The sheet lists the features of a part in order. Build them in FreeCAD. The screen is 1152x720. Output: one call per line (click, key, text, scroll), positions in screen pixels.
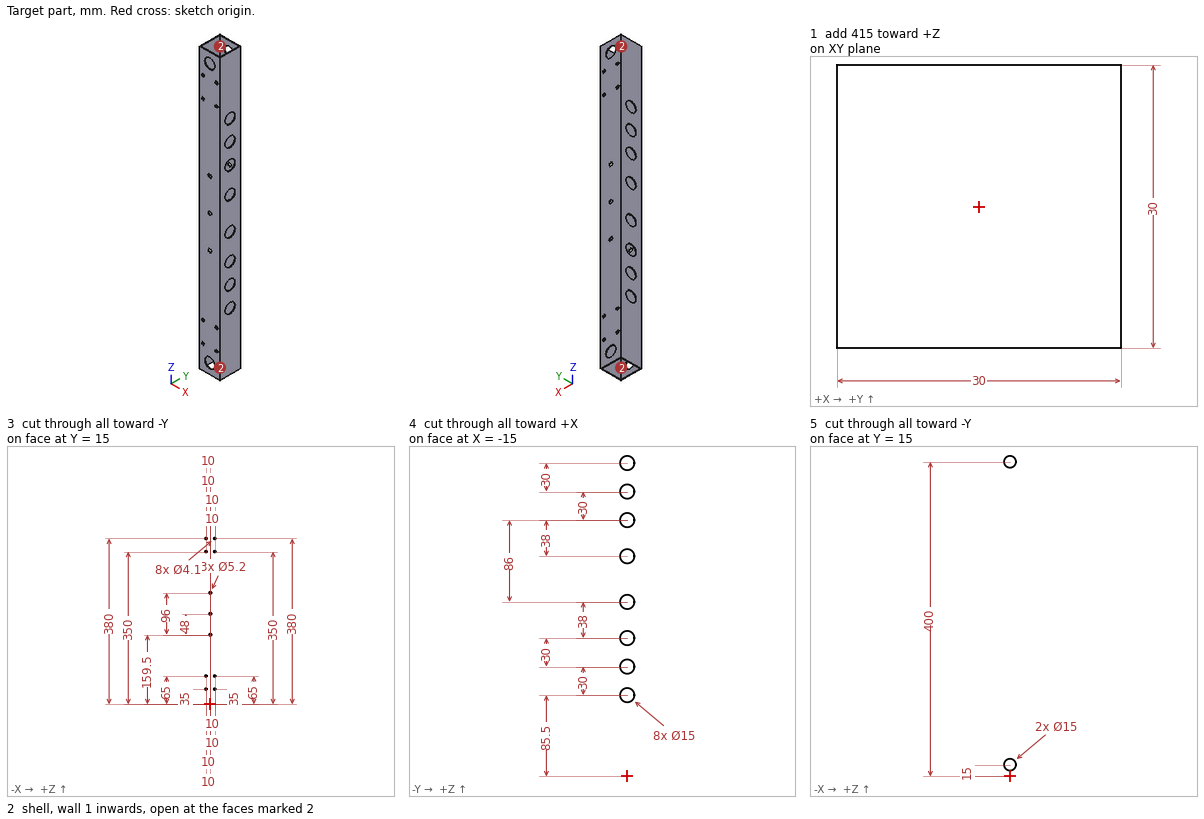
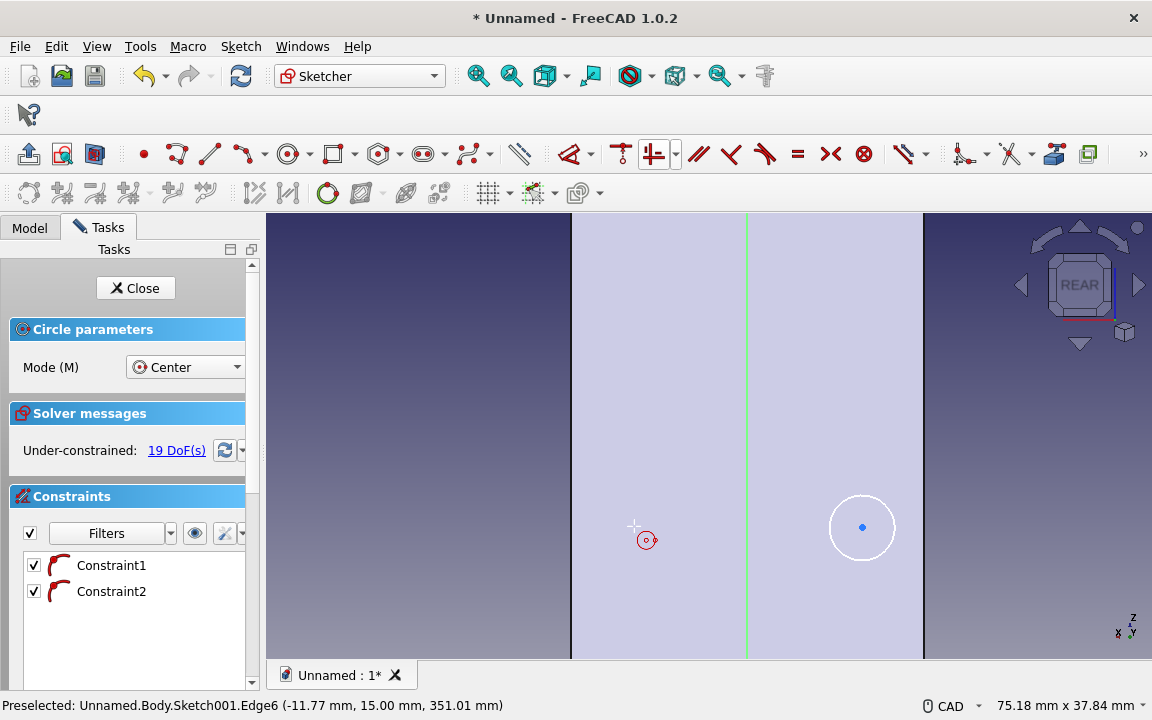
scroll(634, 527, down, 14)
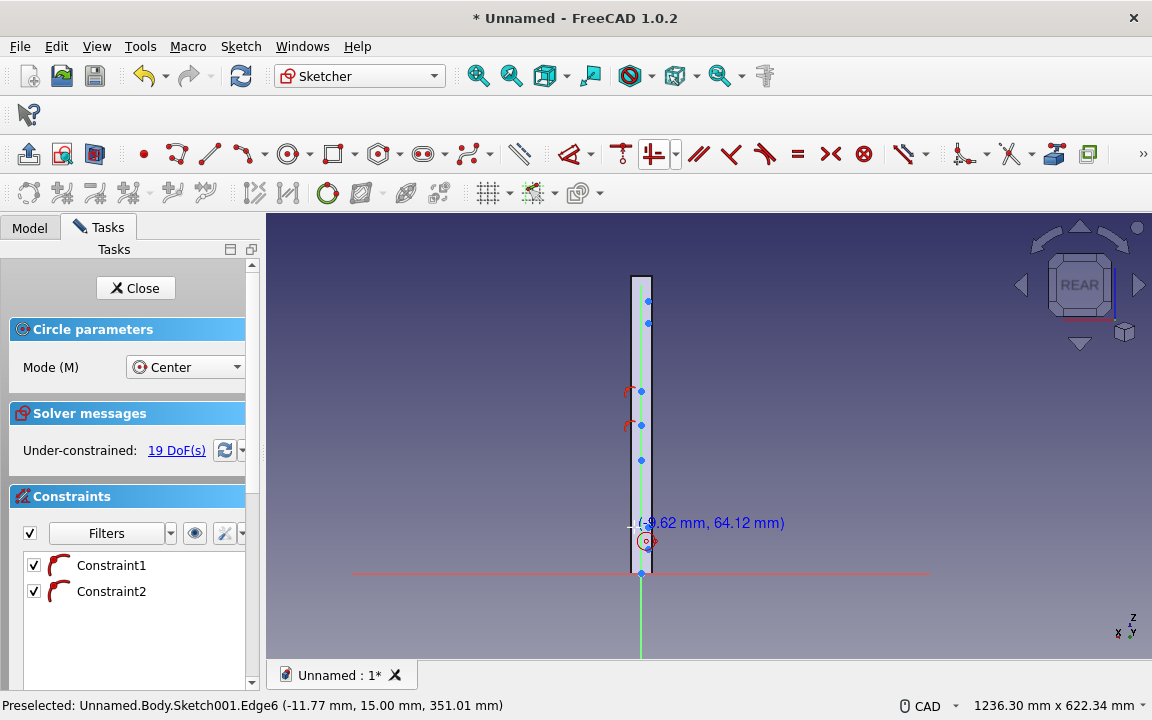
scroll(634, 527, up, 4)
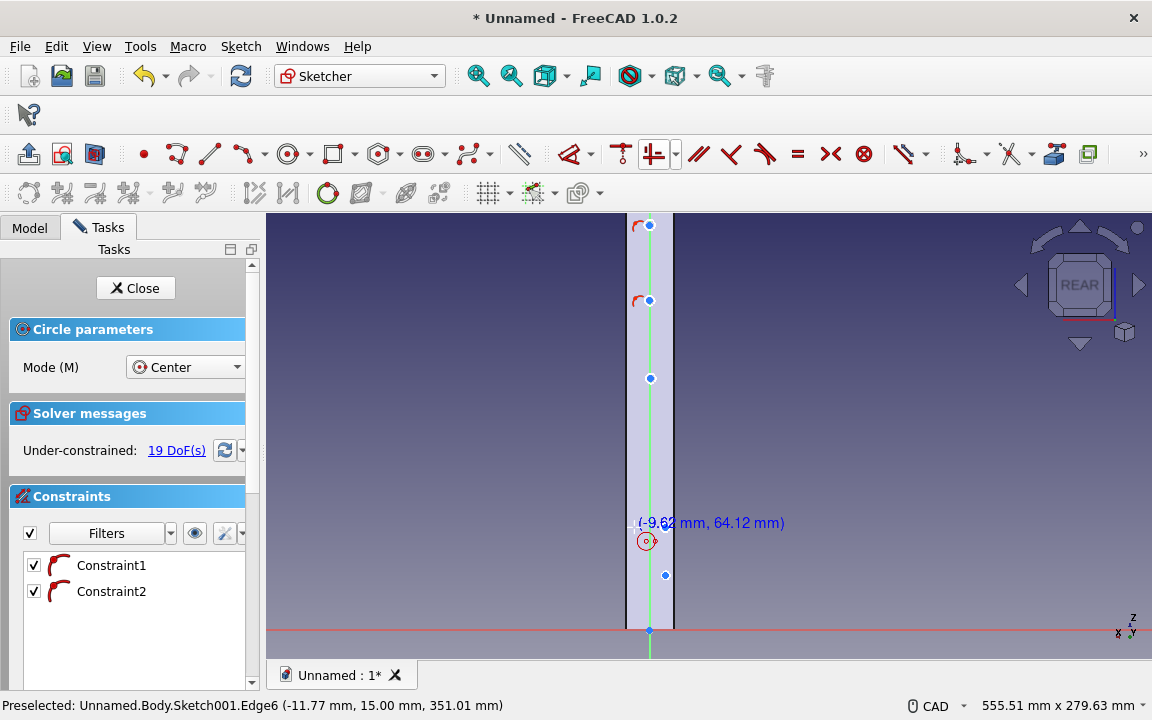
click(634, 526)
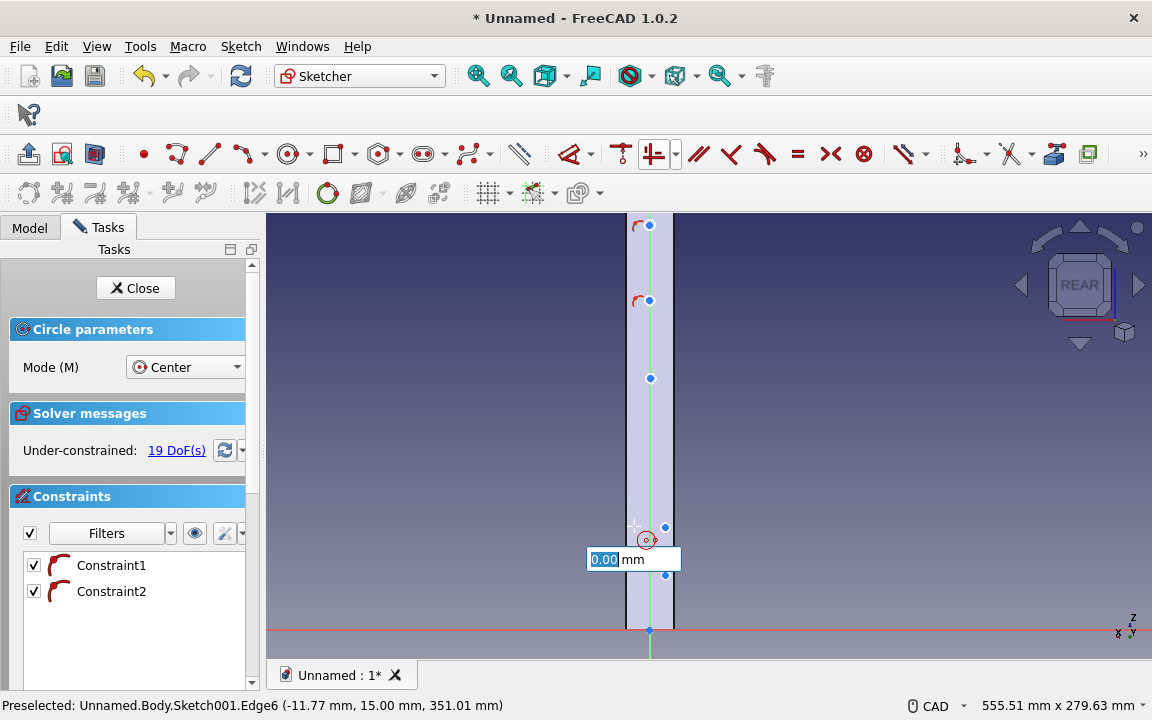
scroll(631, 524, up, 8)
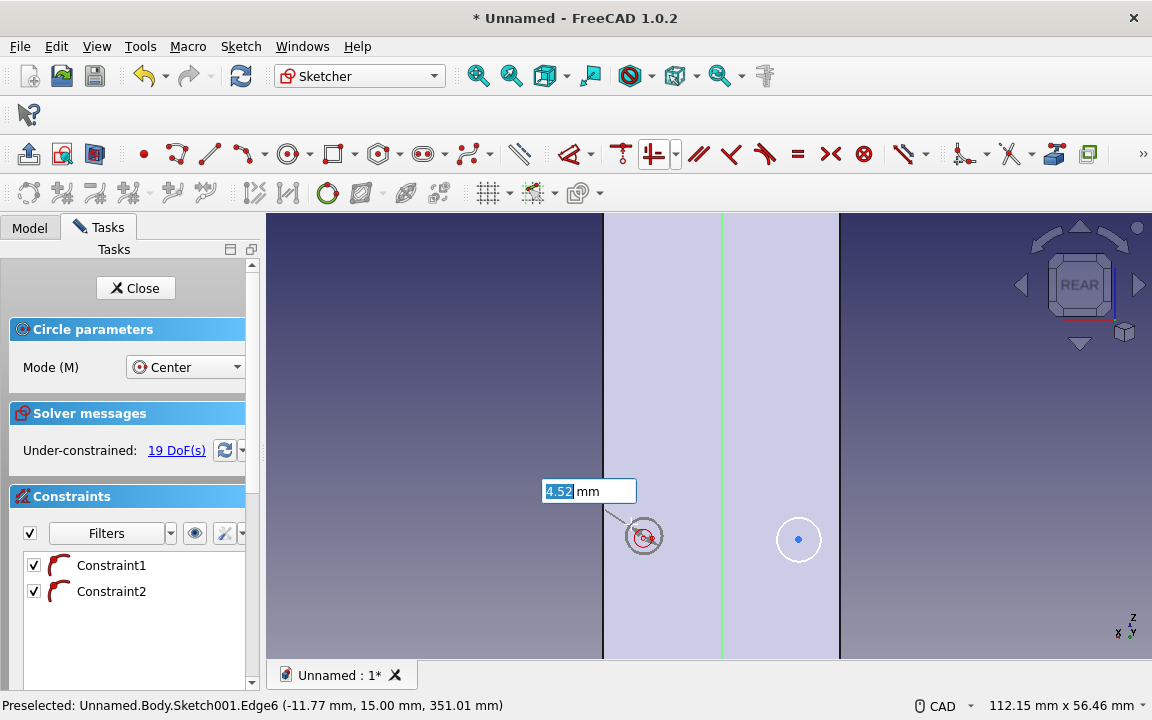
click(632, 521)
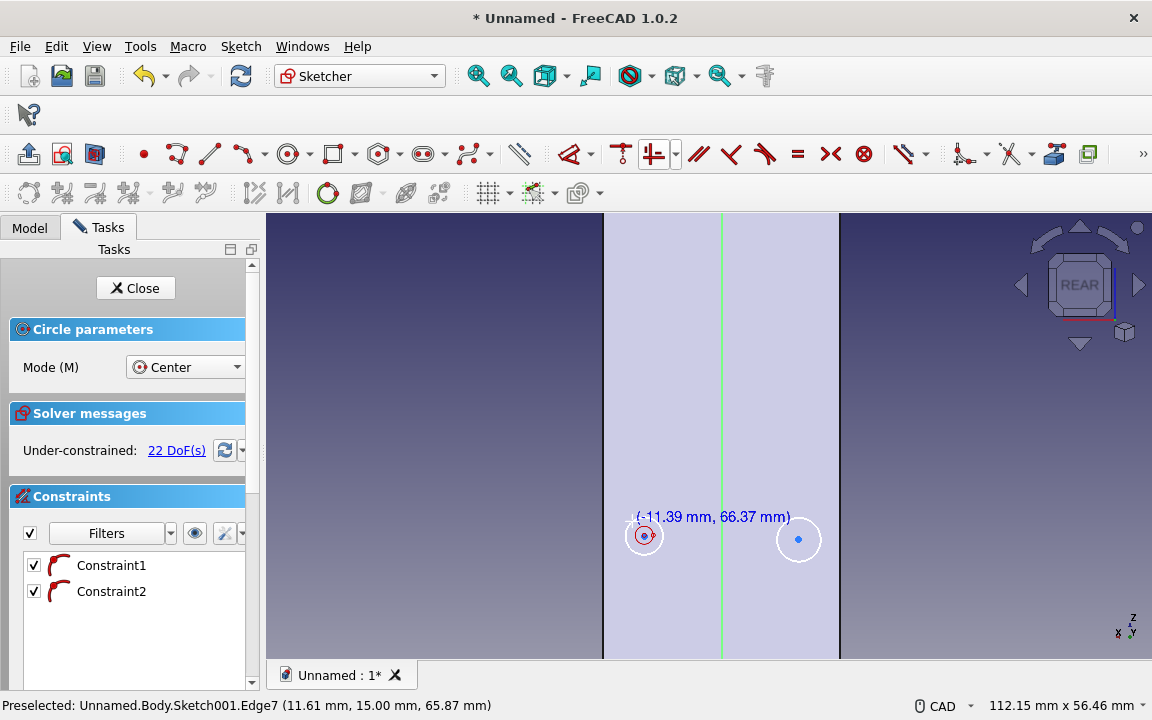
scroll(632, 526, down, 12)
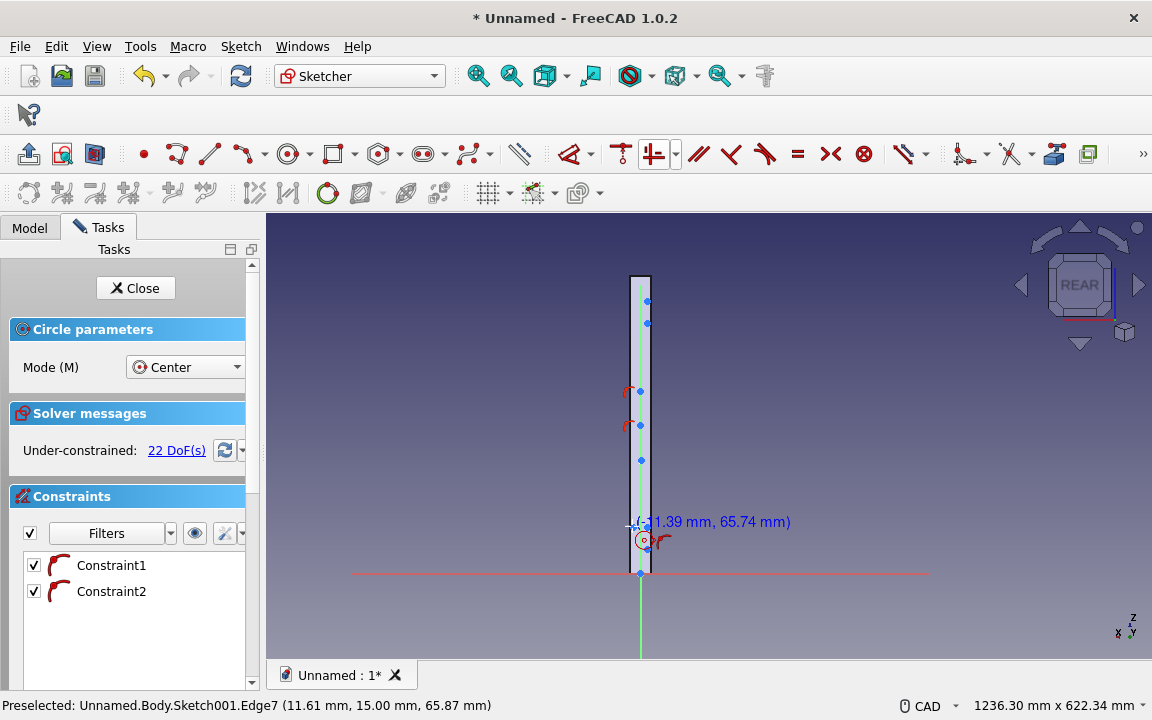
scroll(633, 323, up, 14)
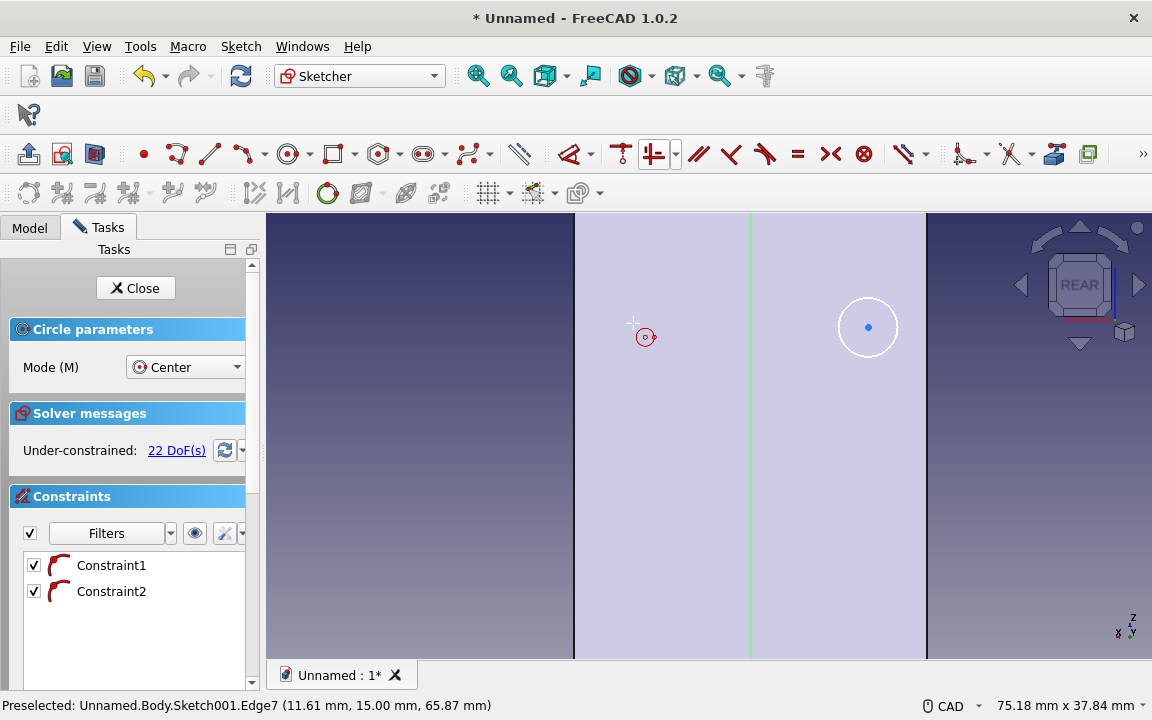
scroll(633, 322, down, 14)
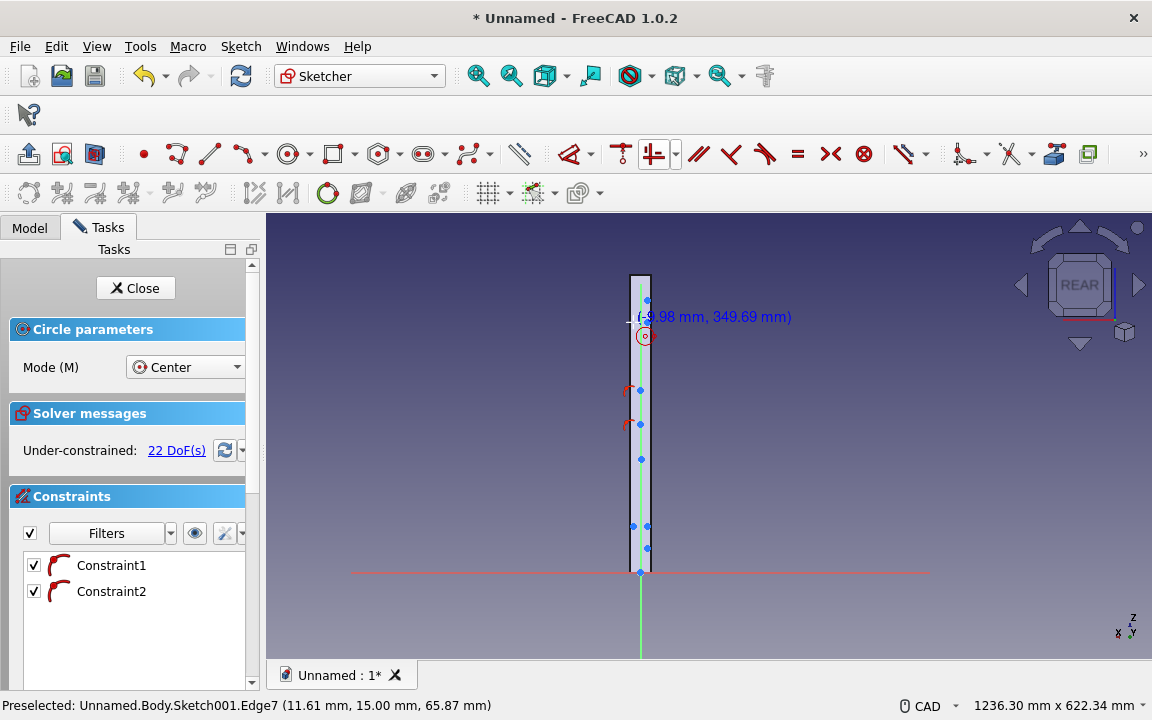
scroll(633, 322, up, 4)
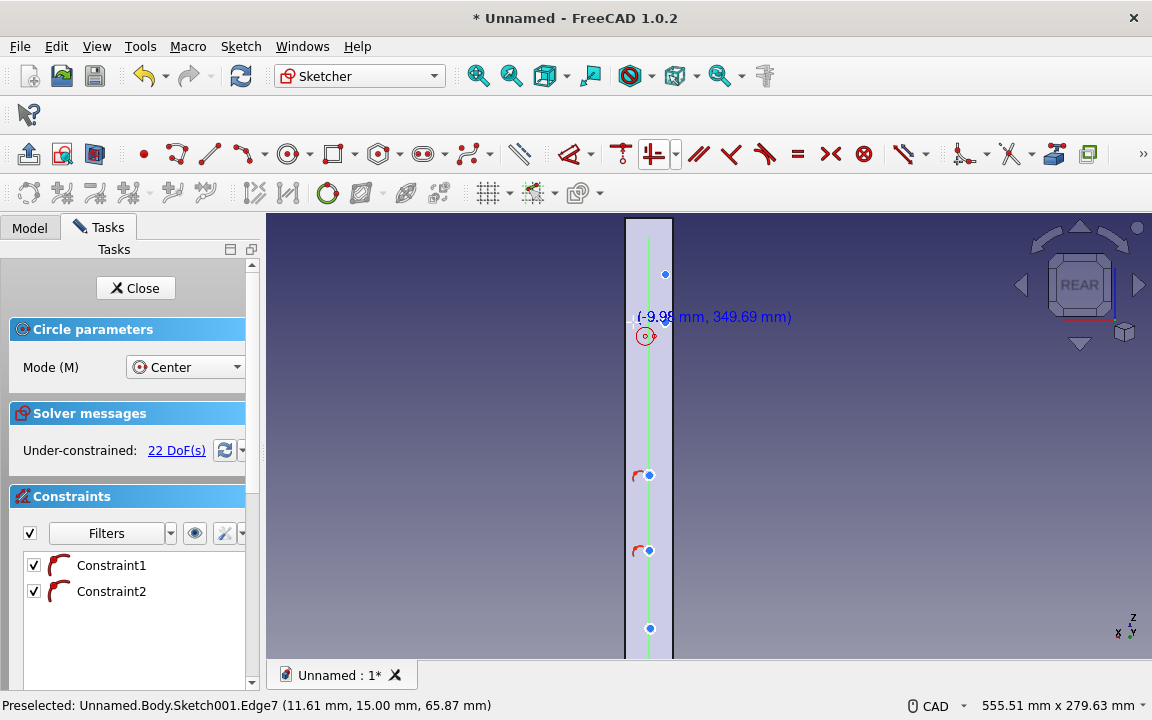
click(633, 322)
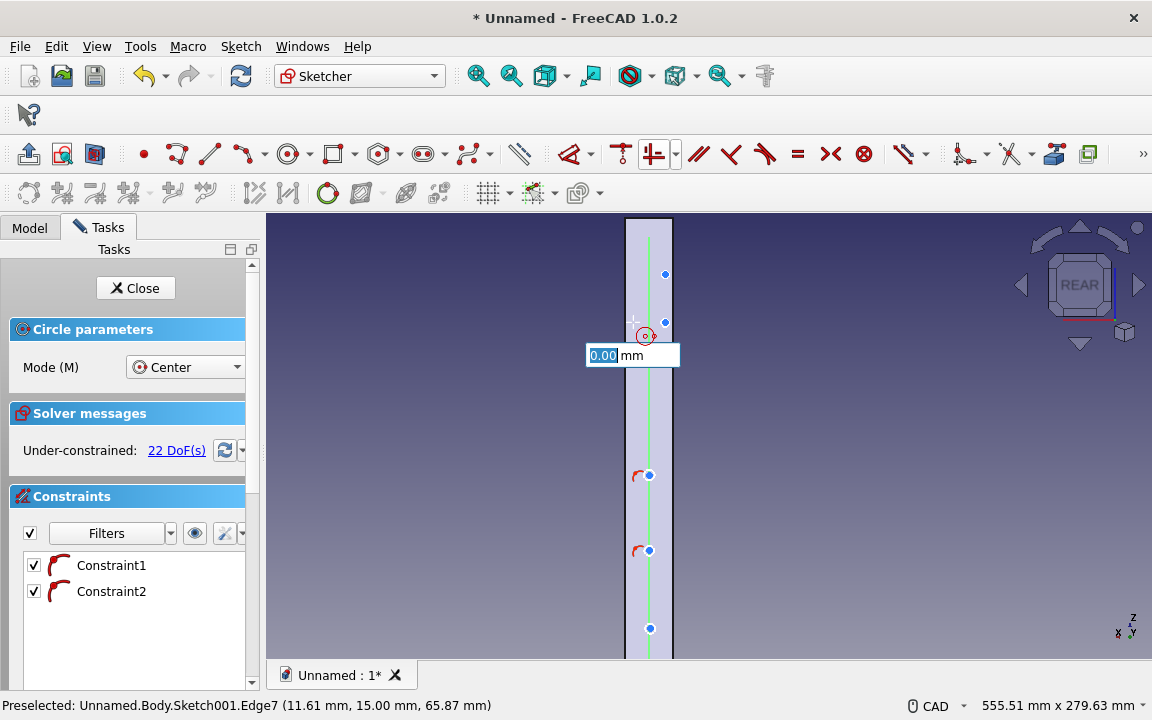
scroll(631, 320, up, 8)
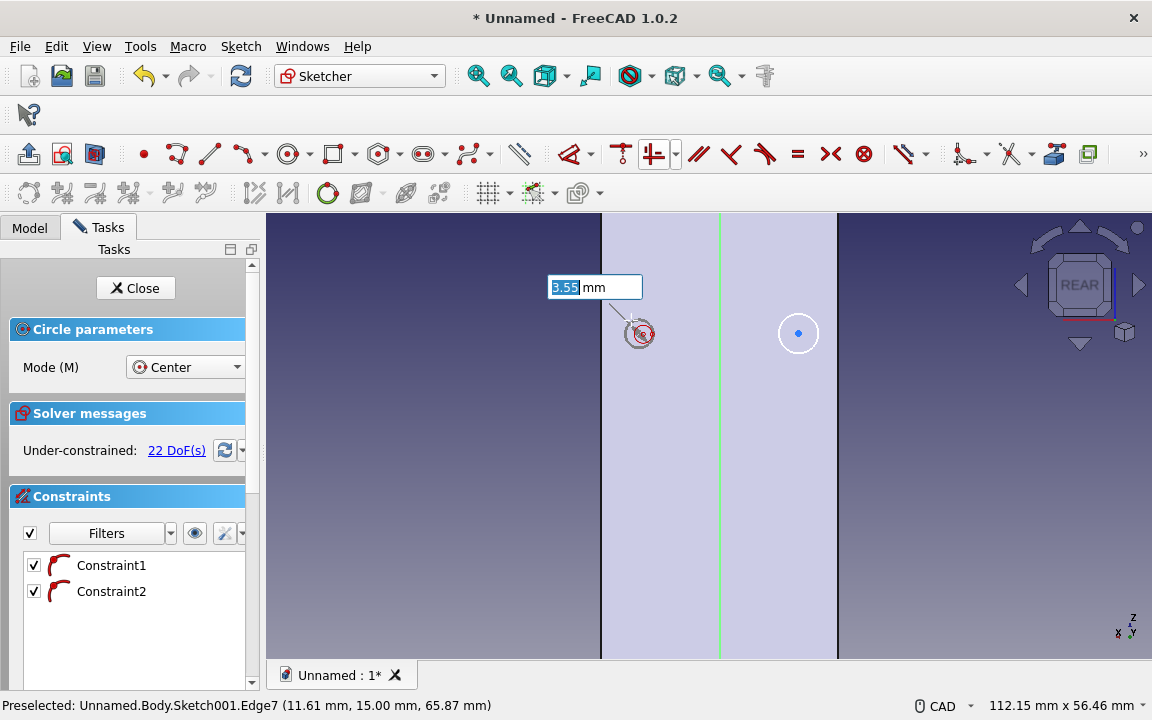
click(629, 317)